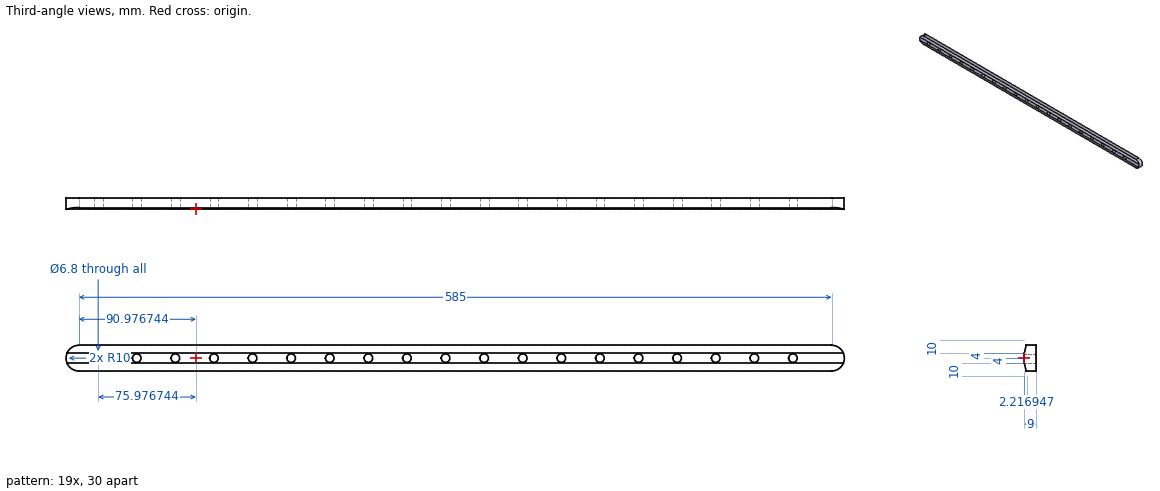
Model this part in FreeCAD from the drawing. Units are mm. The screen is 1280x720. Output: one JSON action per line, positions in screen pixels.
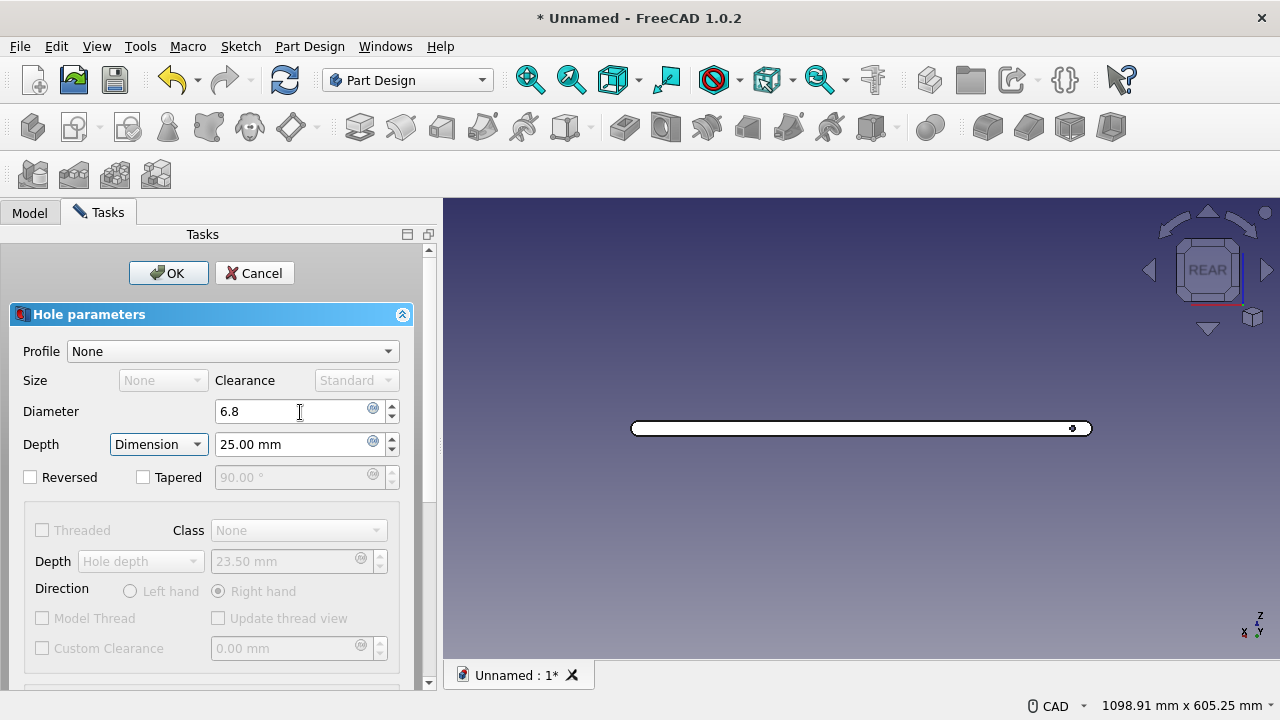
{"action": "left_click", "coordinate": [160, 444]}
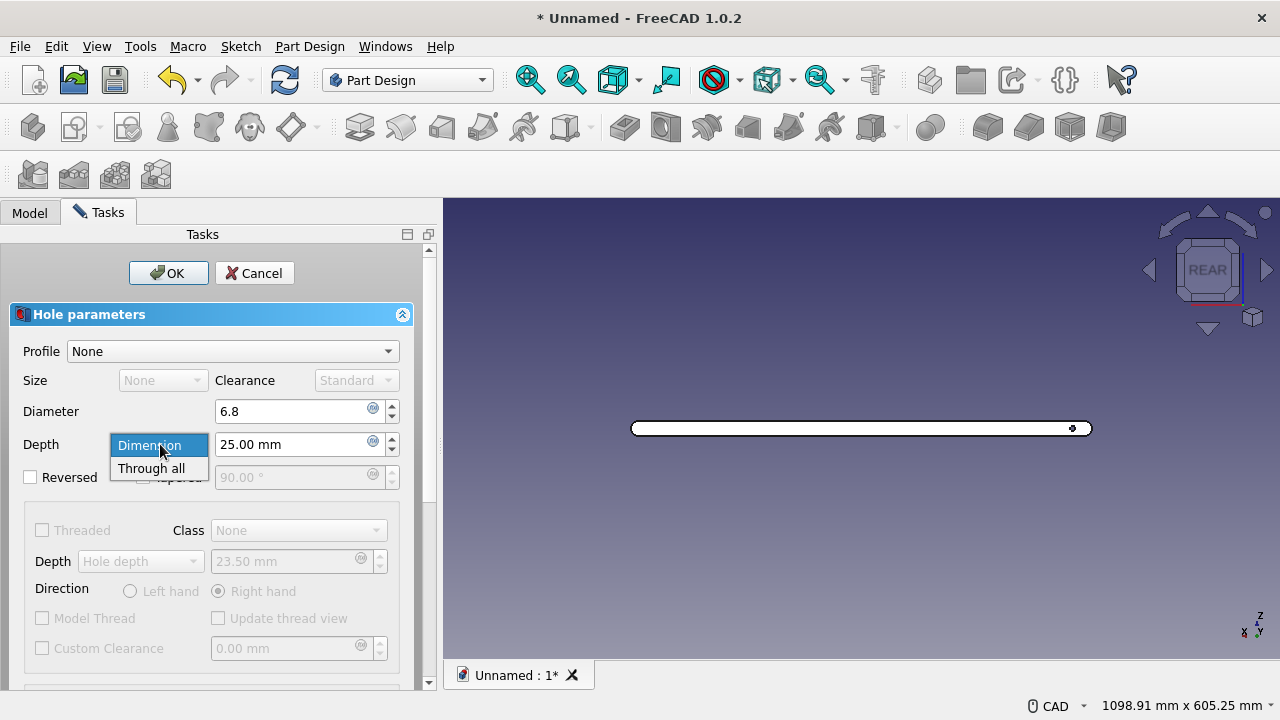
{"action": "left_click", "coordinate": [158, 468]}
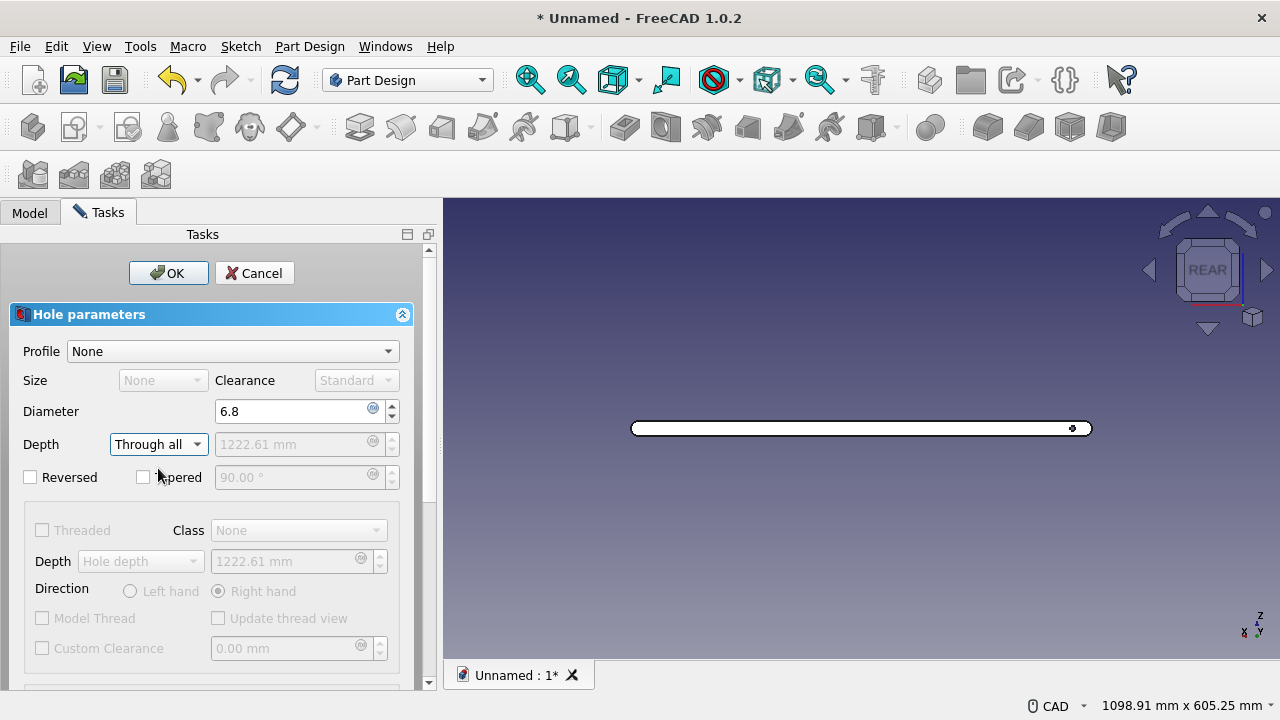
{"action": "left_click", "coordinate": [169, 273]}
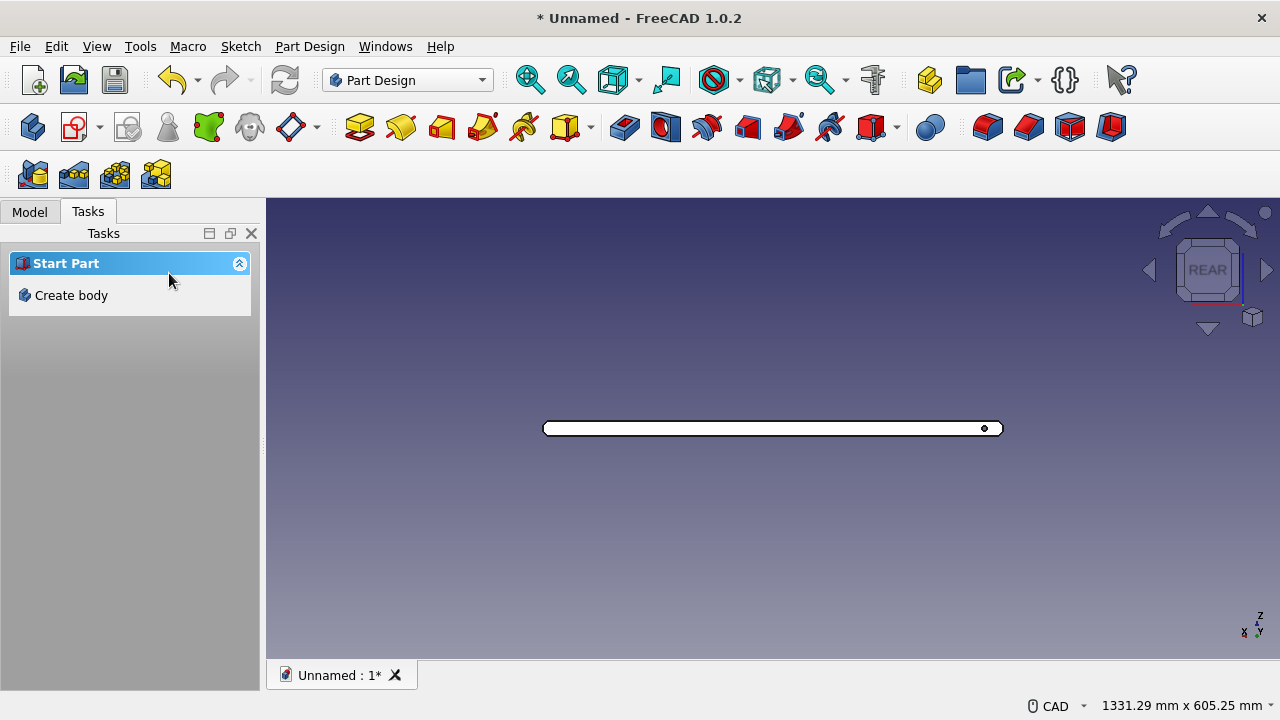
{"action": "left_click", "coordinate": [30, 212]}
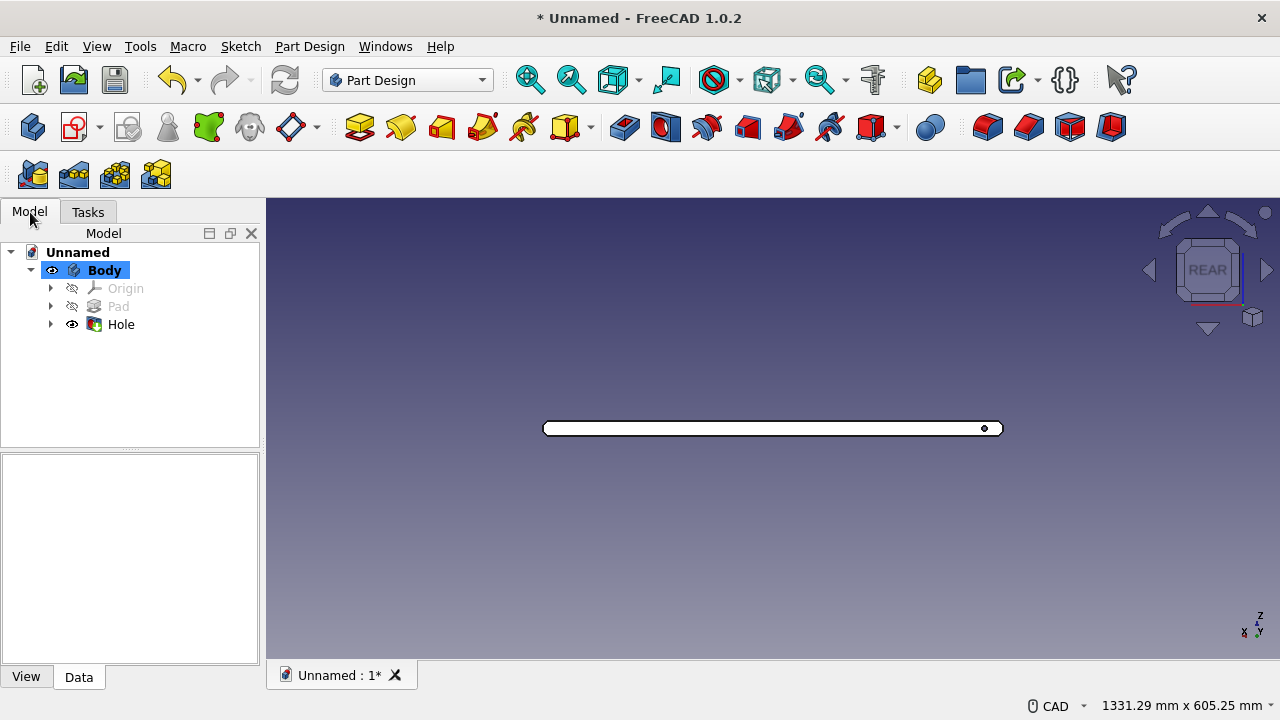
{"action": "left_click", "coordinate": [117, 324]}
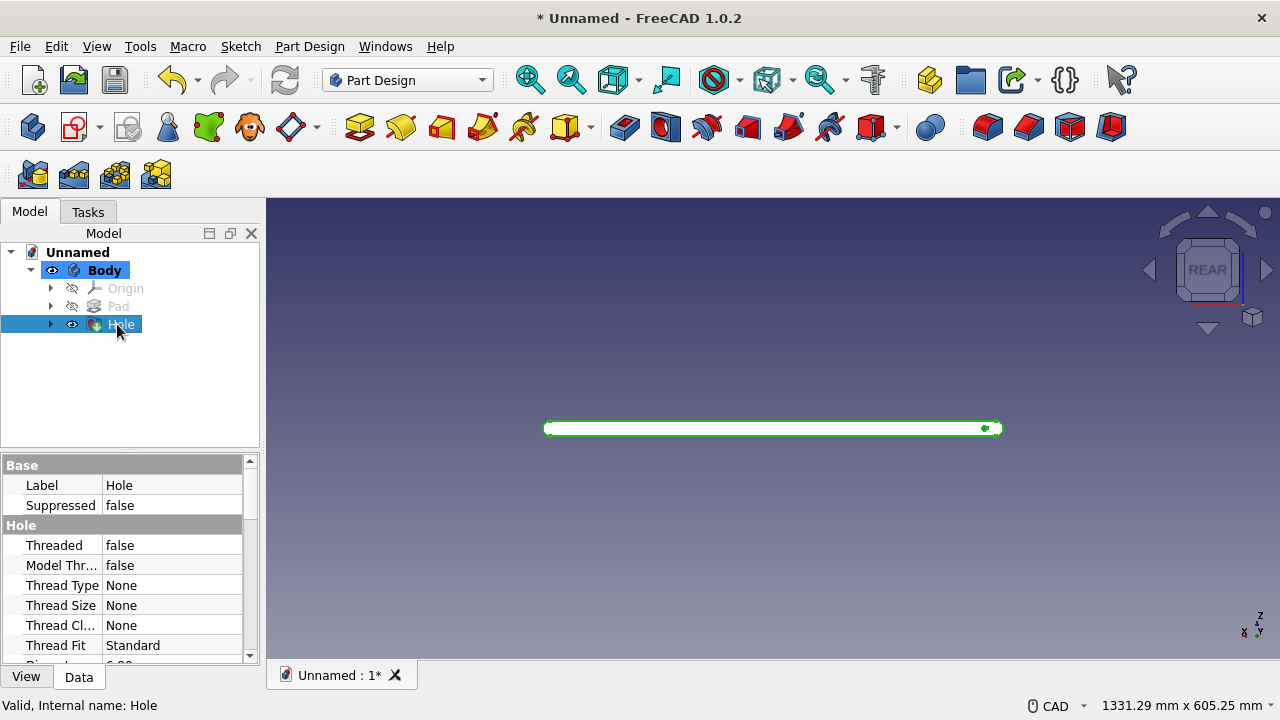
{"action": "left_click", "coordinate": [74, 174]}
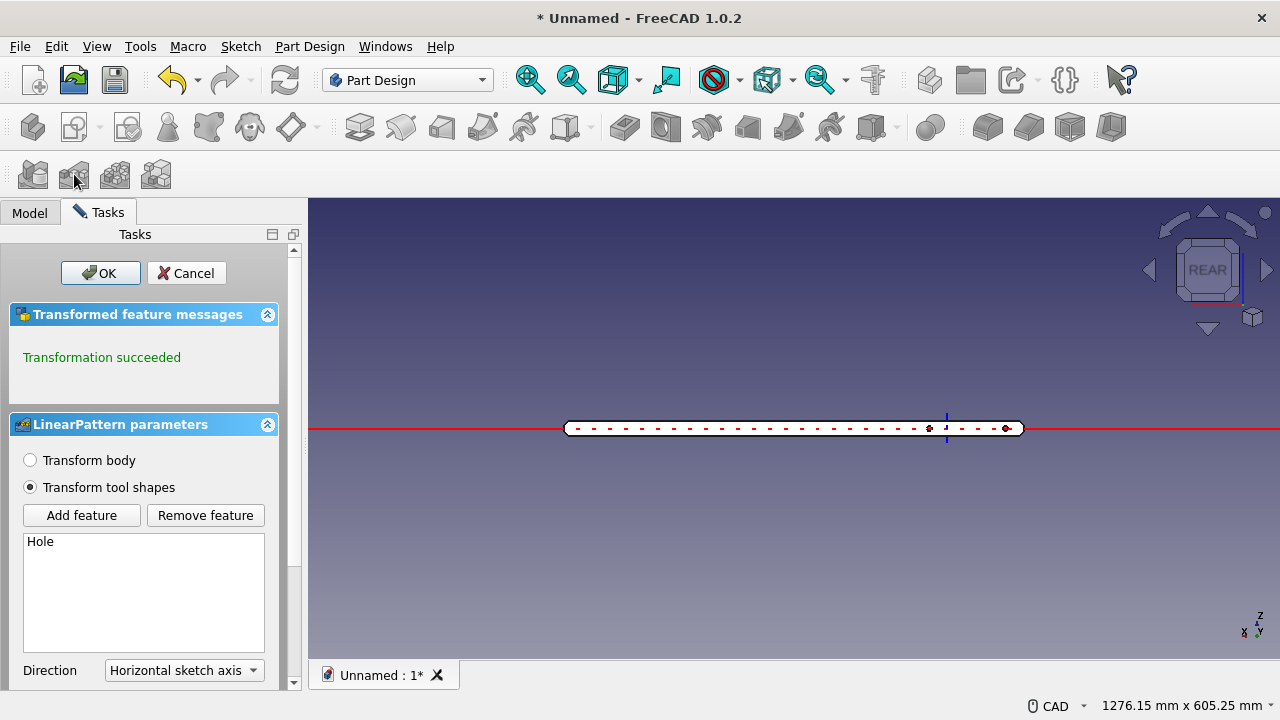
{"action": "left_click", "coordinate": [185, 670]}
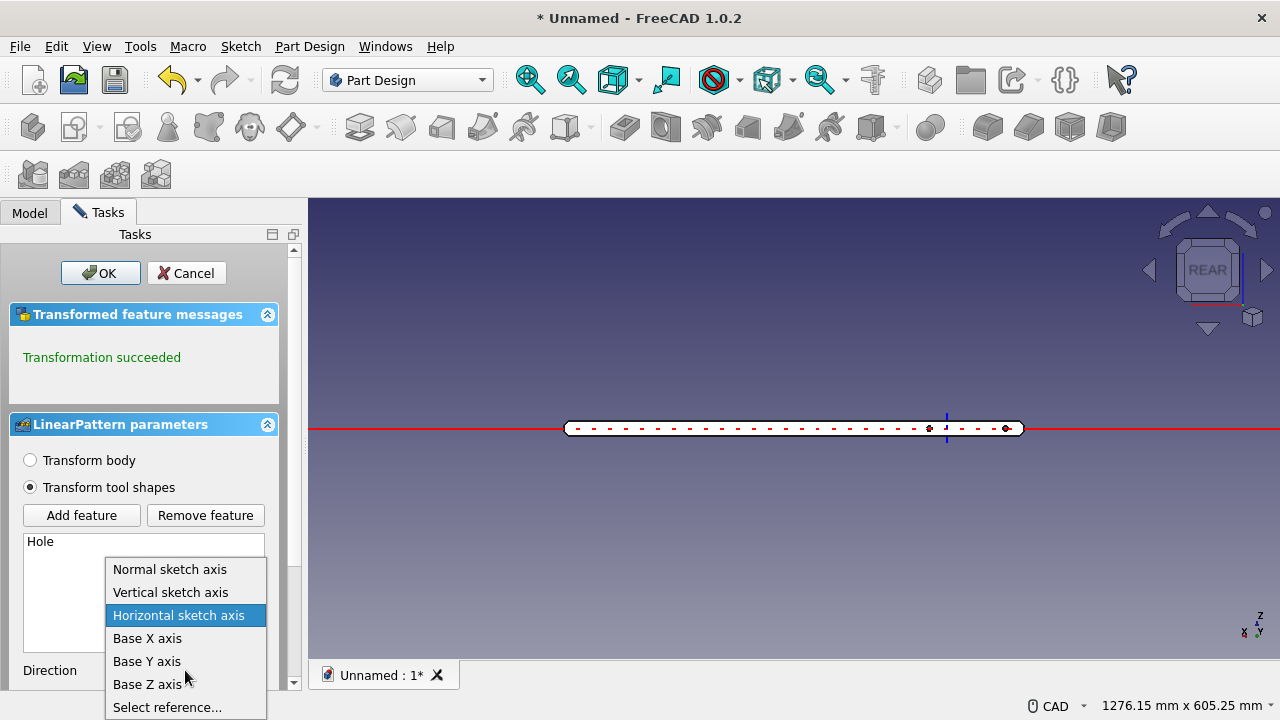
{"action": "left_click", "coordinate": [184, 638]}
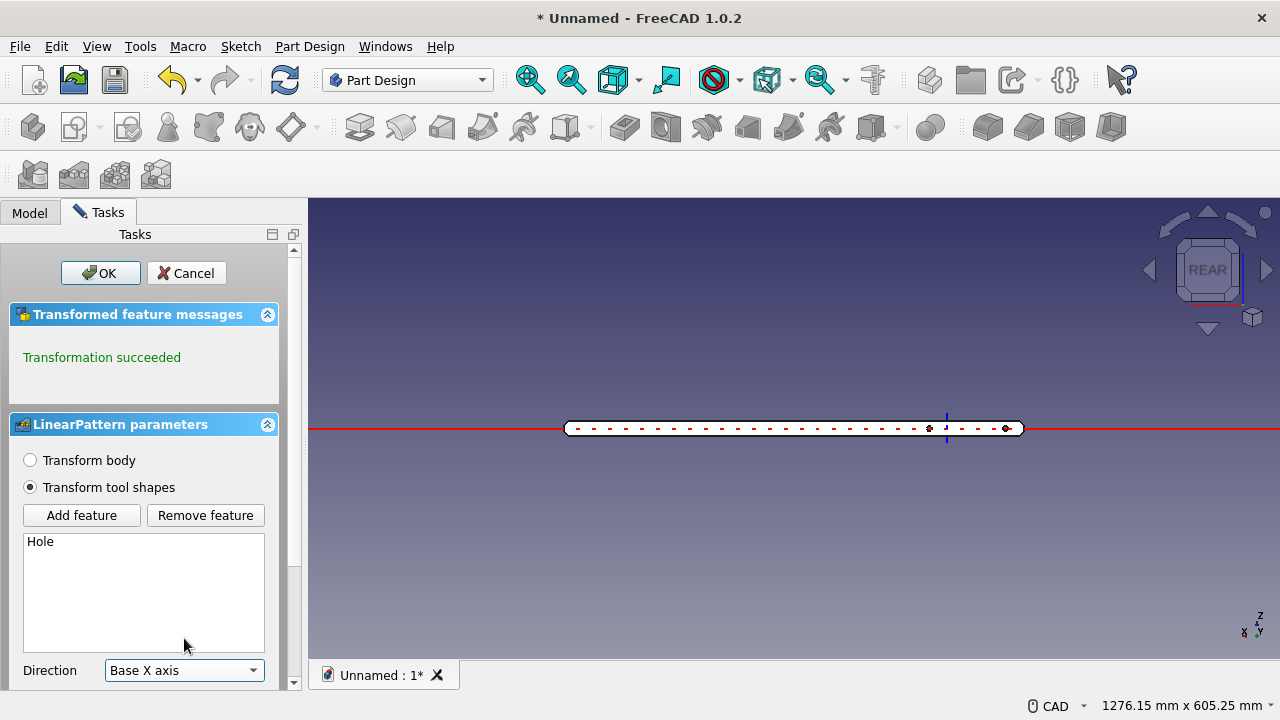
{"action": "scroll", "coordinate": [294, 467], "scroll_direction": "down", "scroll_amount": 2}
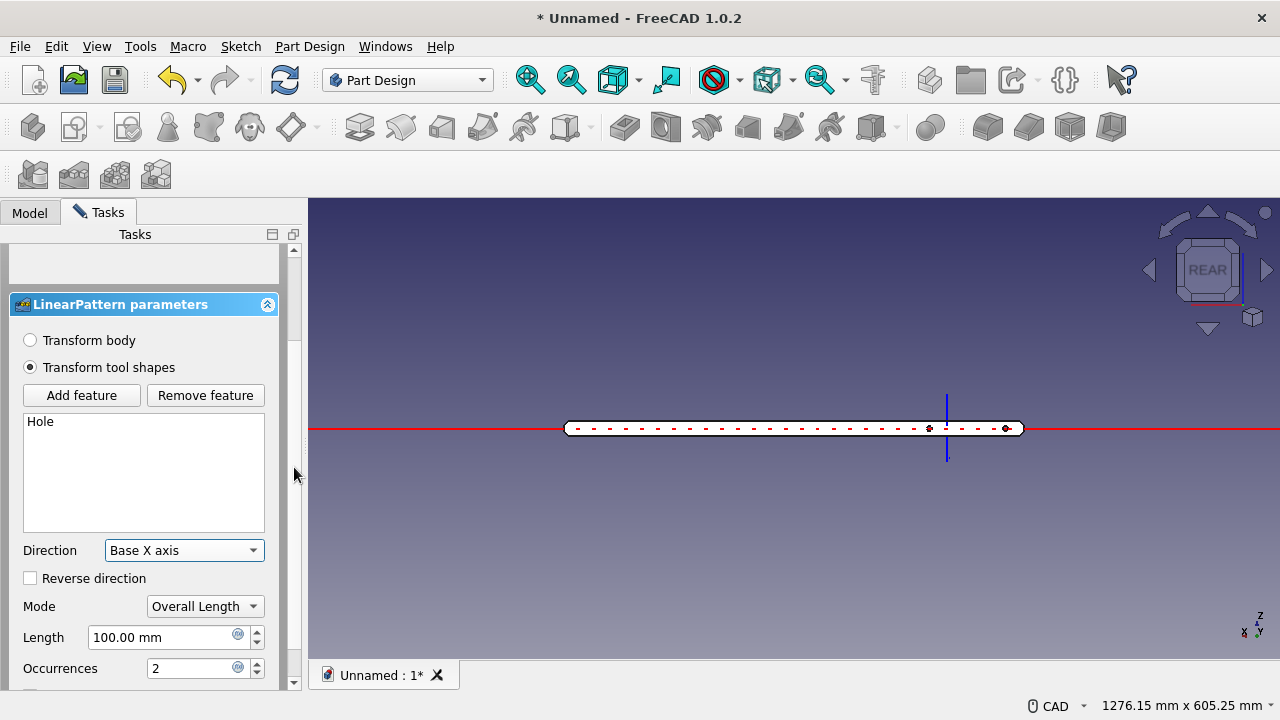
{"action": "left_click", "coordinate": [206, 606]}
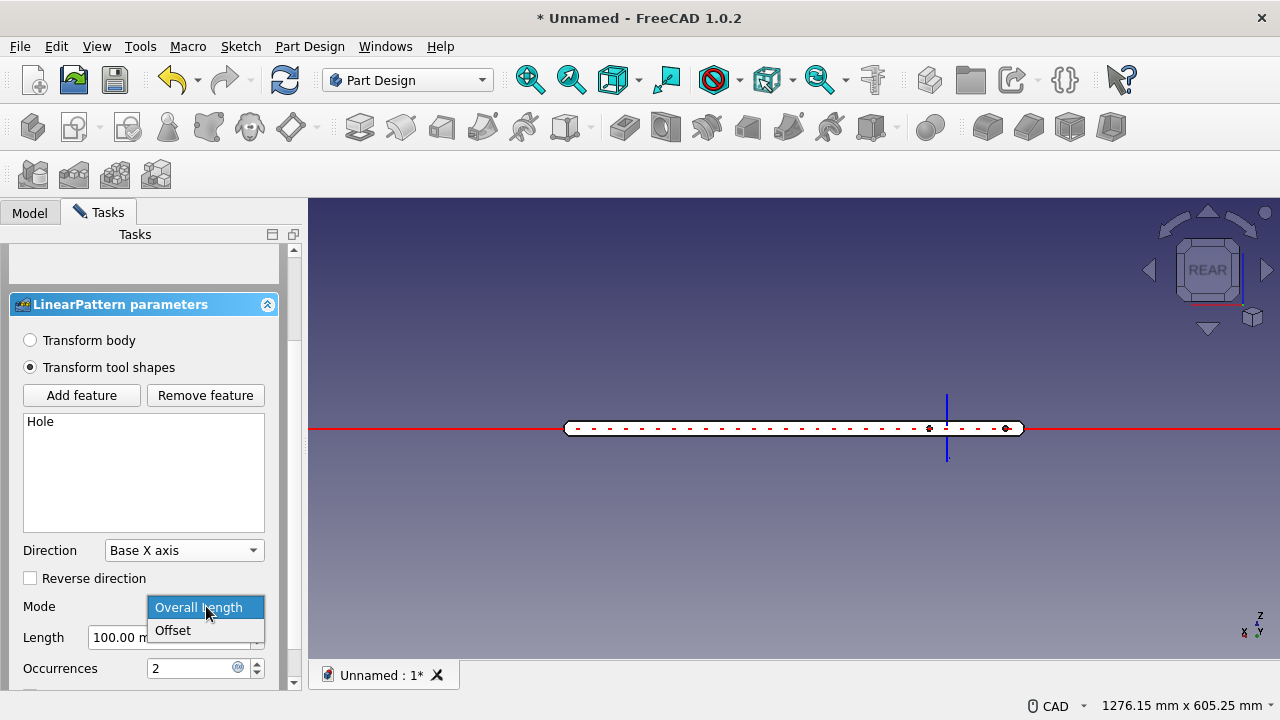
{"action": "left_click", "coordinate": [204, 630]}